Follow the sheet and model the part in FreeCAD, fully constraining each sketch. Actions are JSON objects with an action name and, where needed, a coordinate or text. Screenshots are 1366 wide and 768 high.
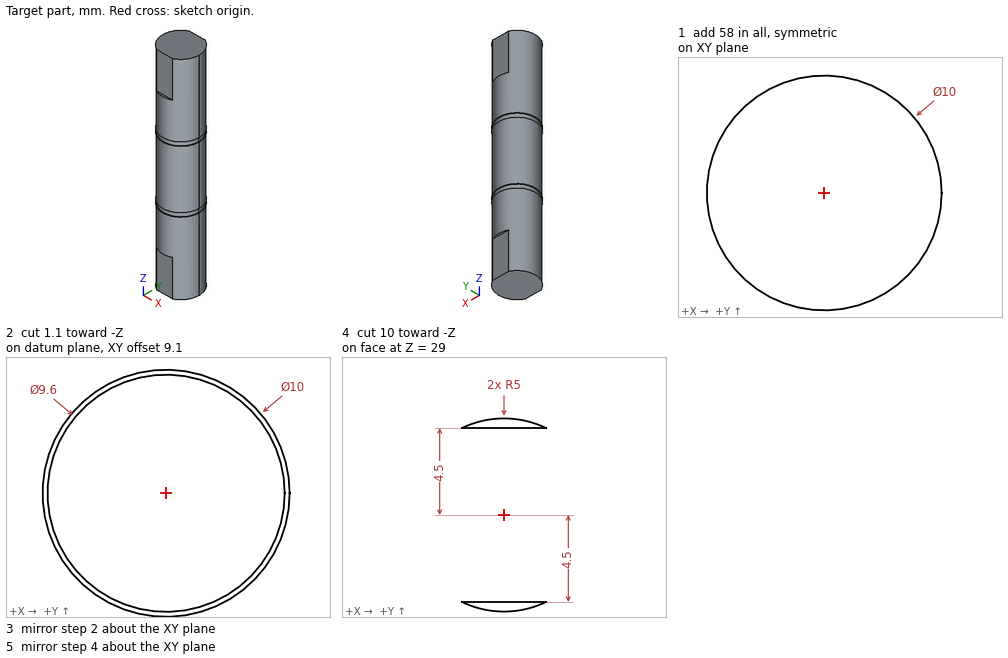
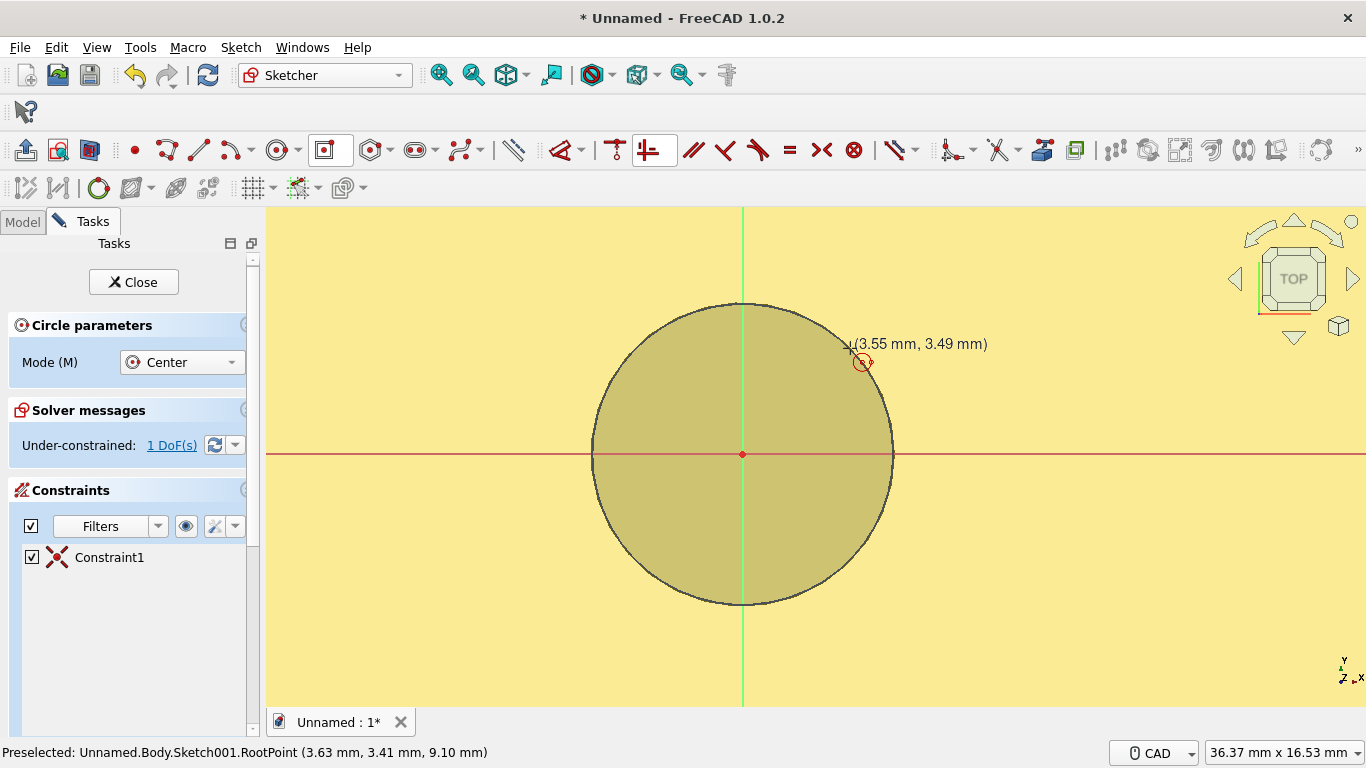
{"action": "left_click", "coordinate": [743, 454]}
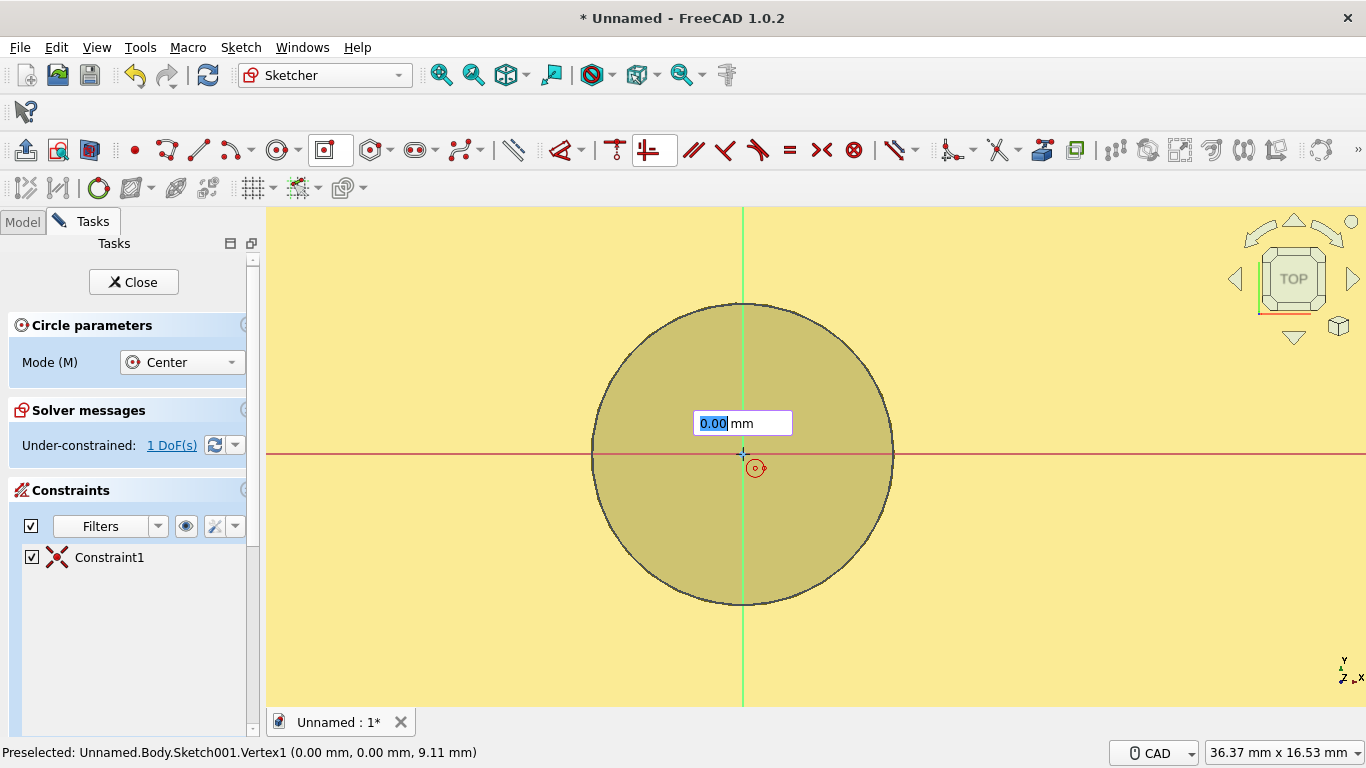
{"action": "scroll", "coordinate": [845, 352], "scroll_direction": "up", "scroll_amount": 5}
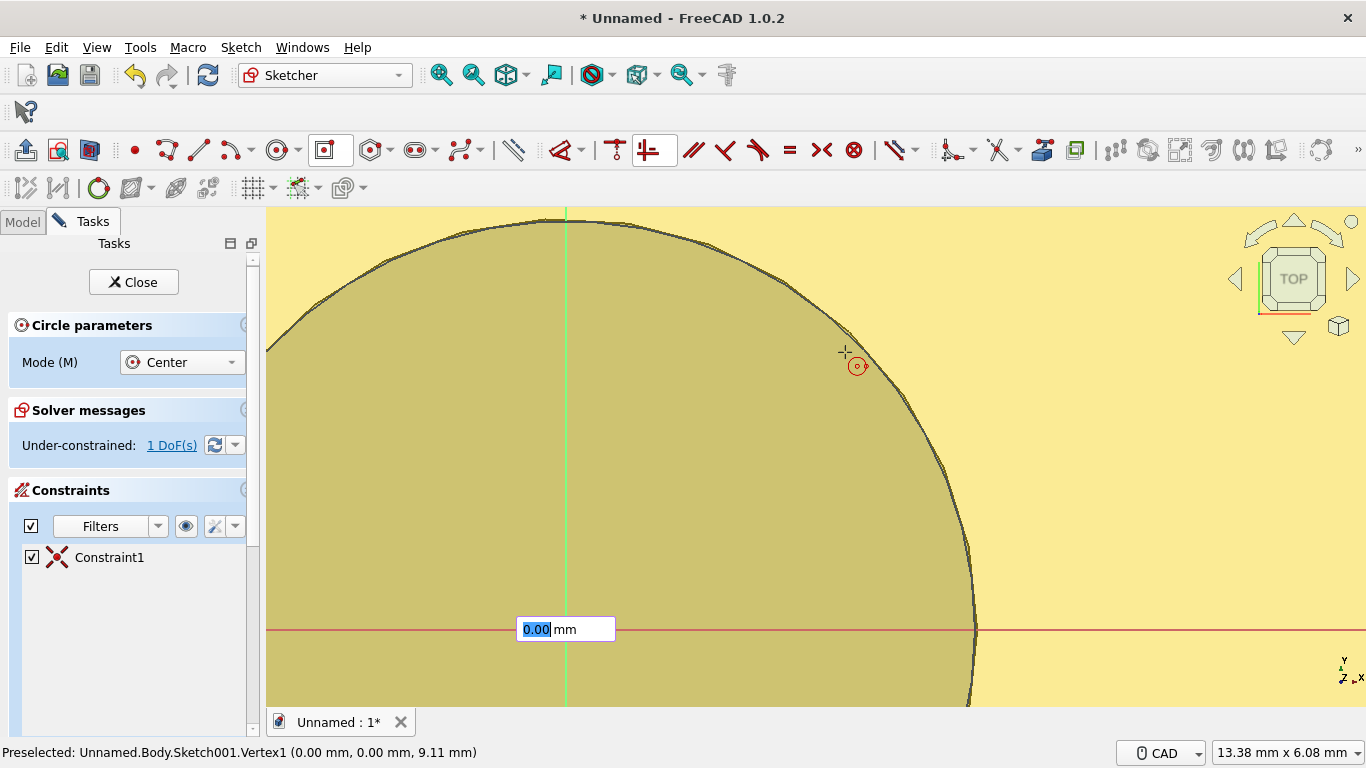
{"action": "left_click", "coordinate": [845, 351]}
{"action": "key", "text": "Escape"}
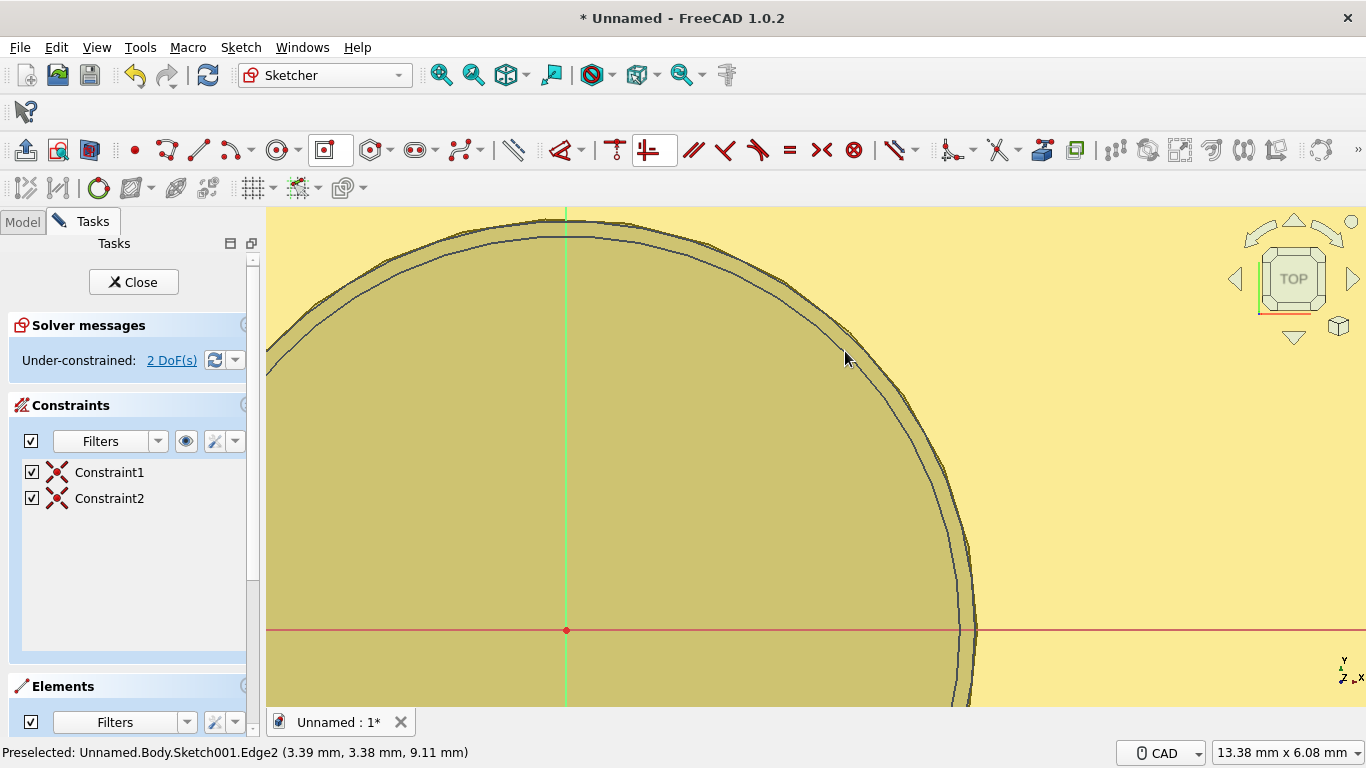
{"action": "key", "text": "d"}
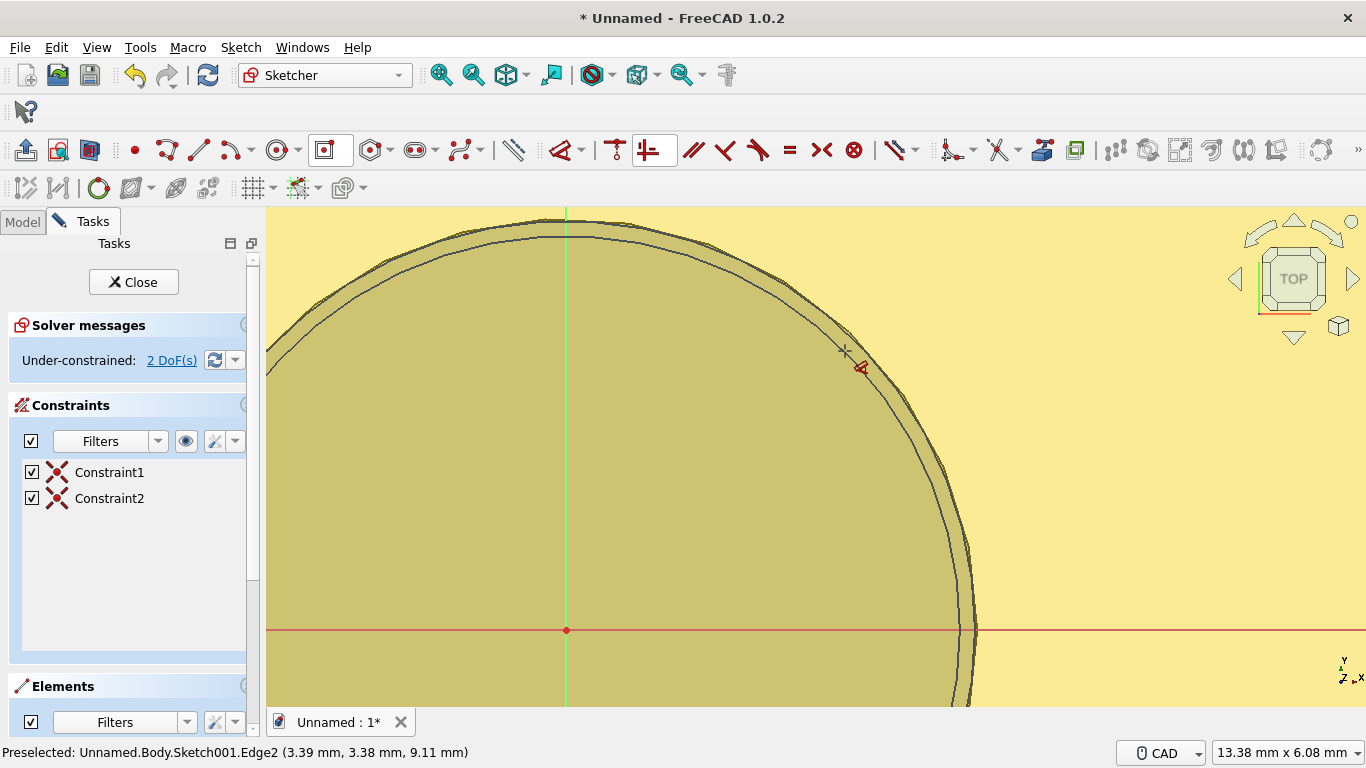
{"action": "left_click", "coordinate": [854, 340]}
{"action": "left_click", "coordinate": [877, 317]}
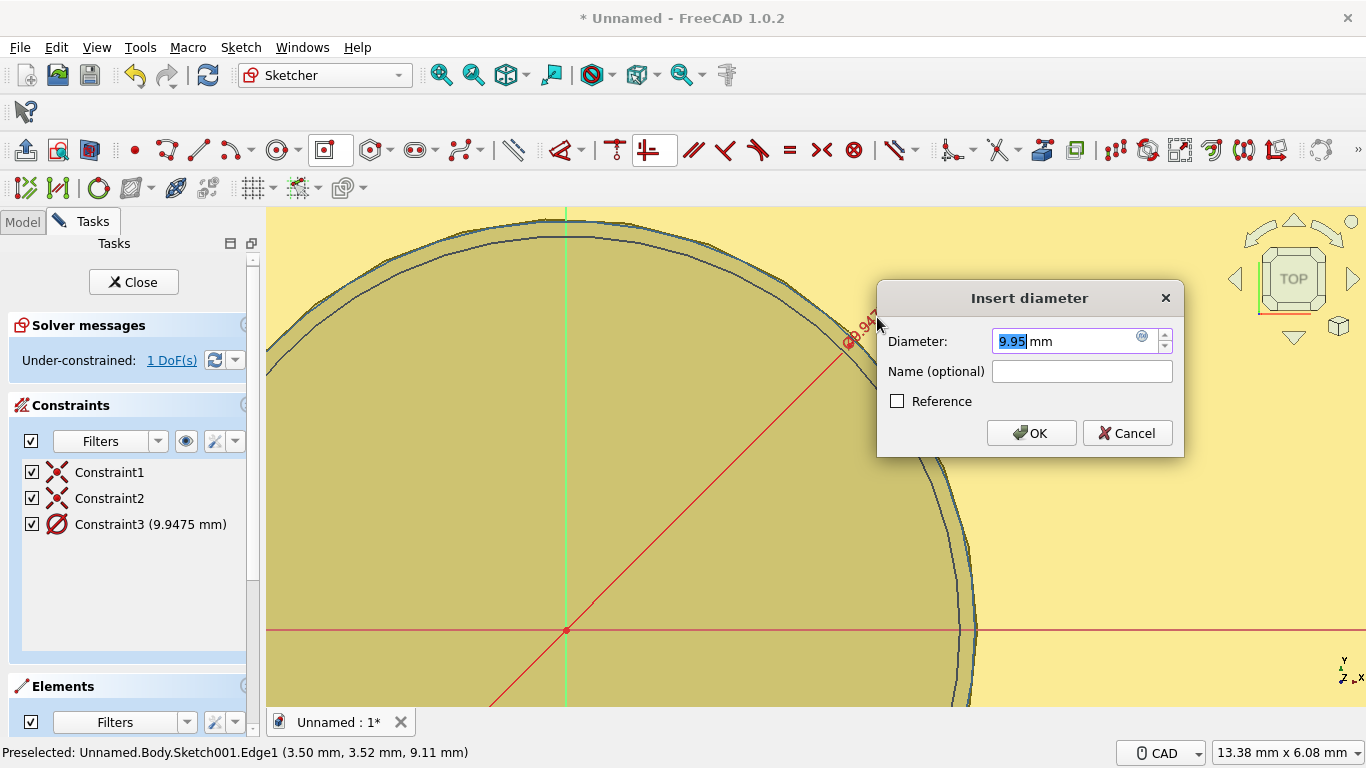
{"action": "type", "text": "10"}
{"action": "key", "text": "Return"}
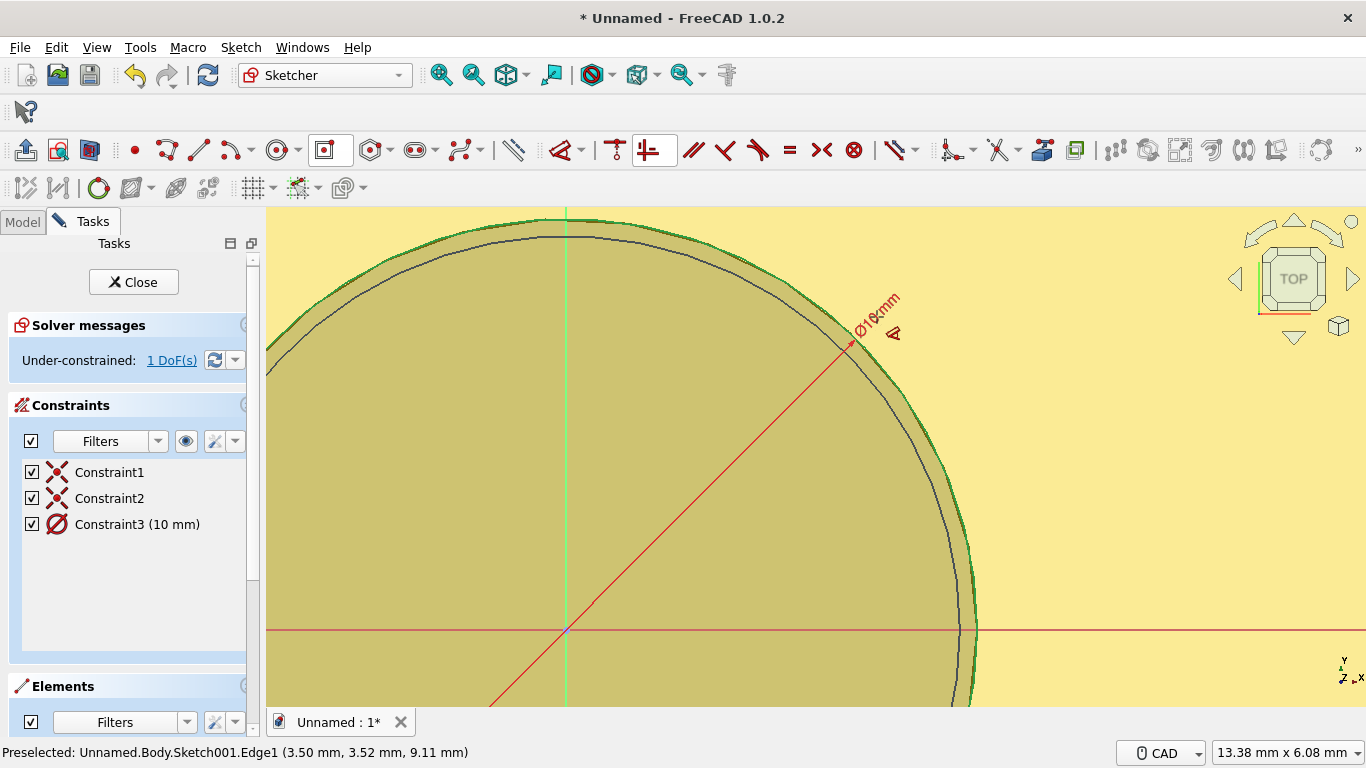
{"action": "left_click", "coordinate": [844, 351]}
{"action": "left_click", "coordinate": [974, 509]}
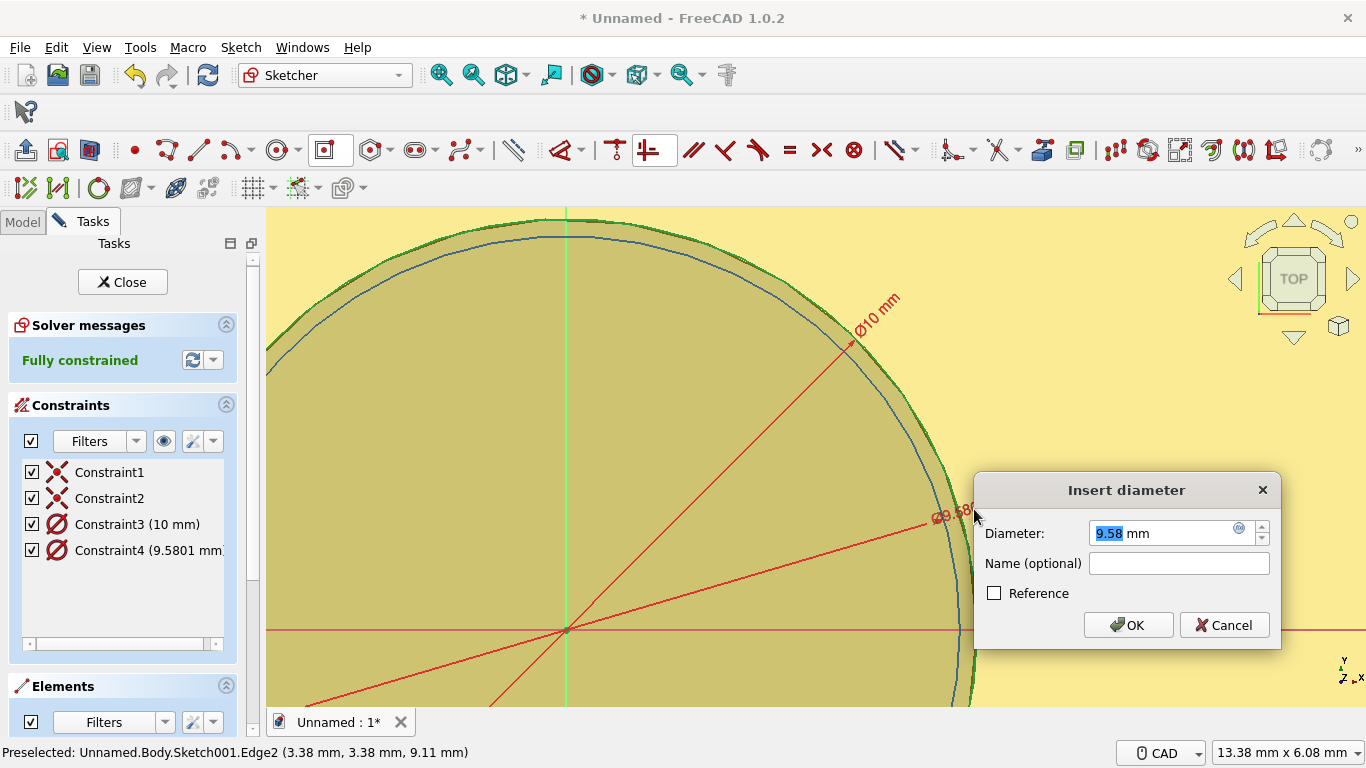
{"action": "type", "text": "9.6"}
{"action": "key", "text": "Return"}
{"action": "key", "text": "Escape"}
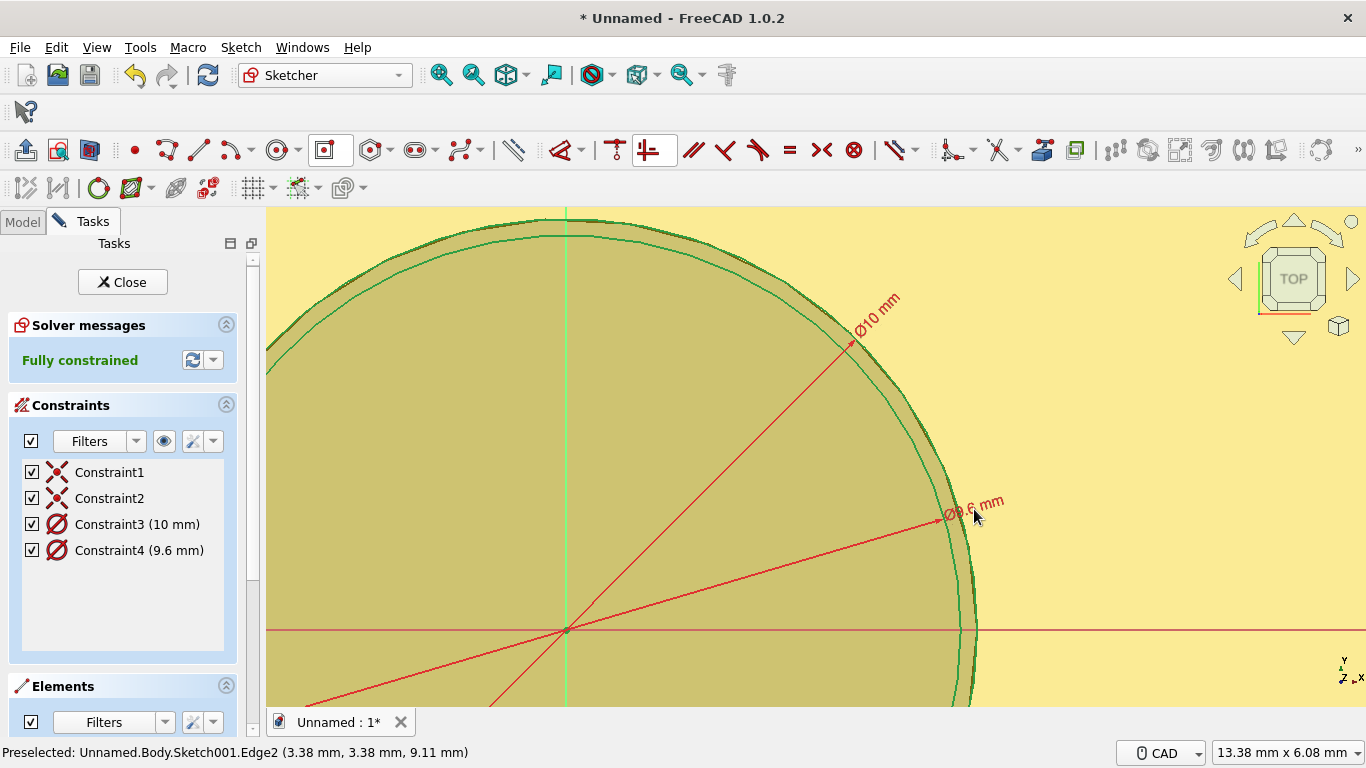
{"action": "left_click", "coordinate": [123, 282]}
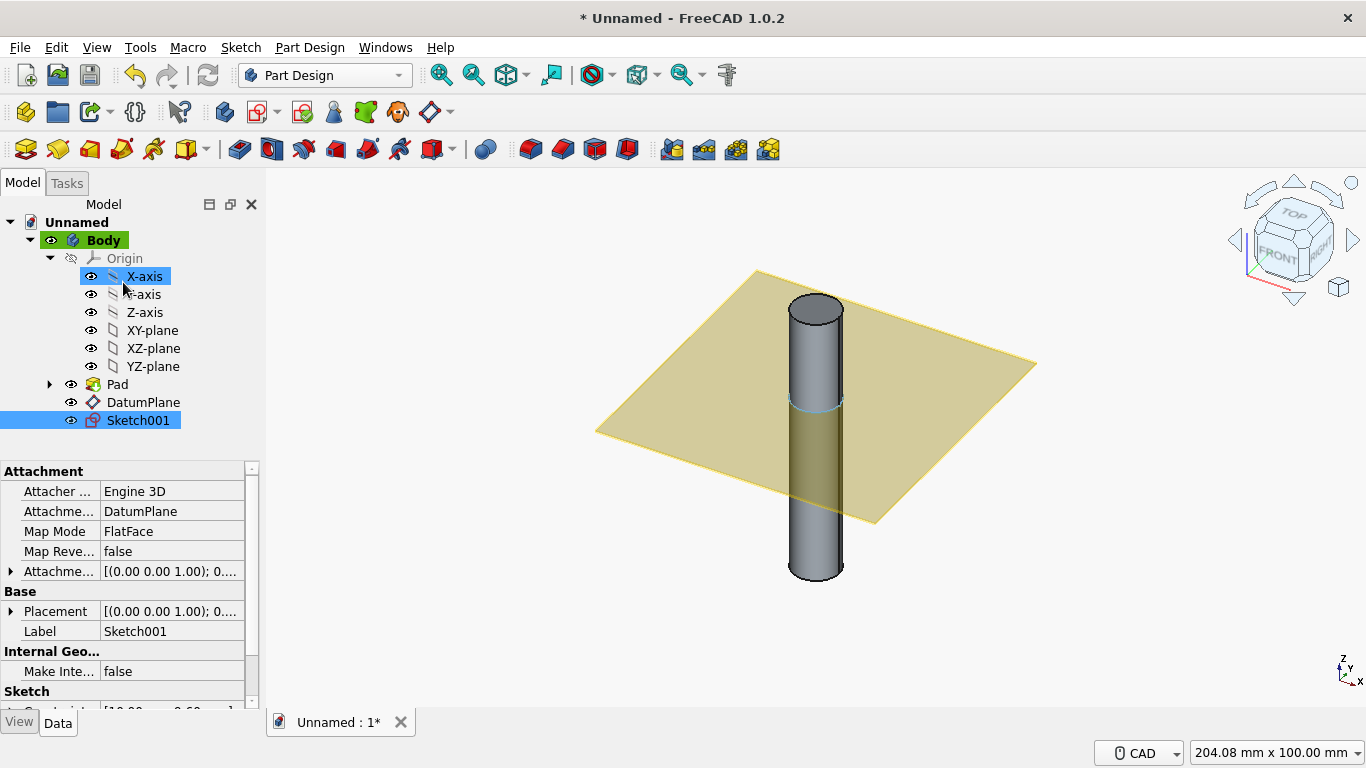
{"action": "left_click", "coordinate": [240, 150]}